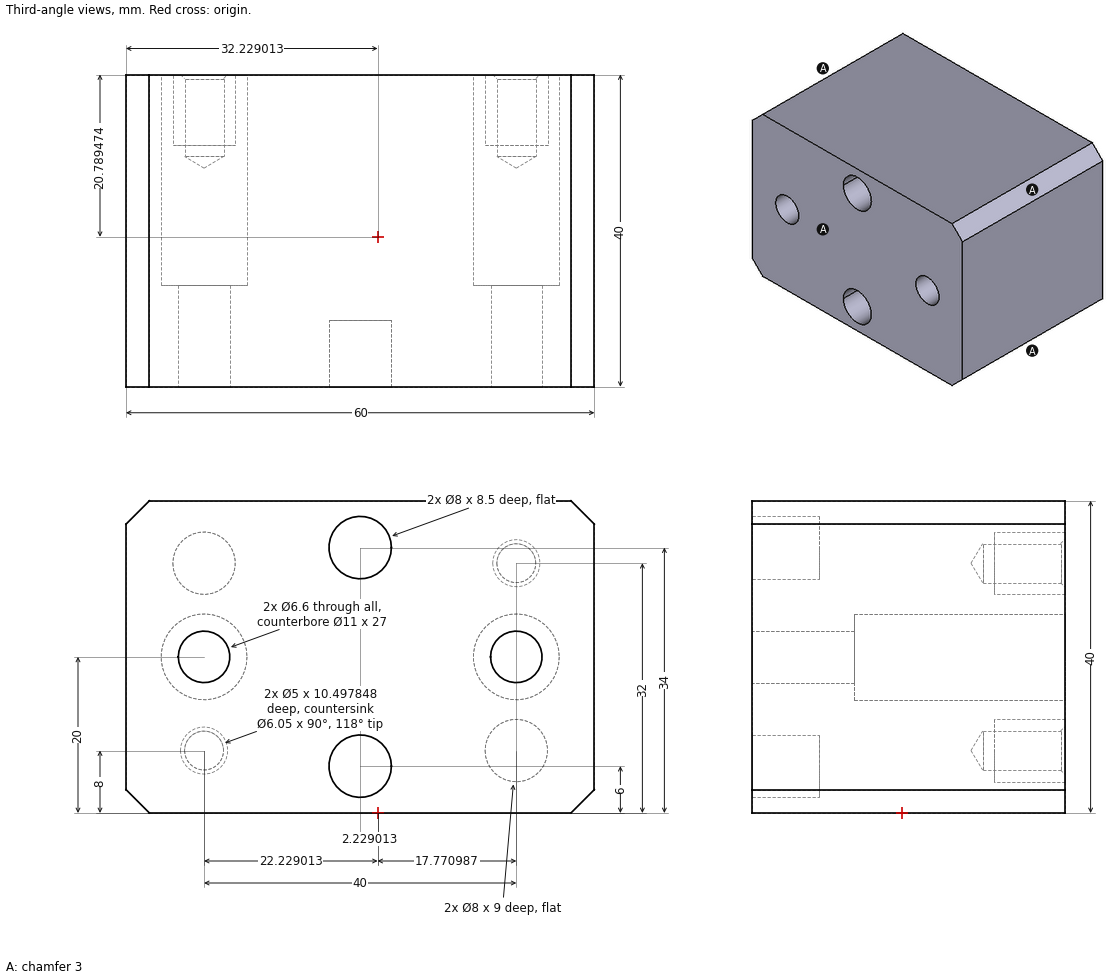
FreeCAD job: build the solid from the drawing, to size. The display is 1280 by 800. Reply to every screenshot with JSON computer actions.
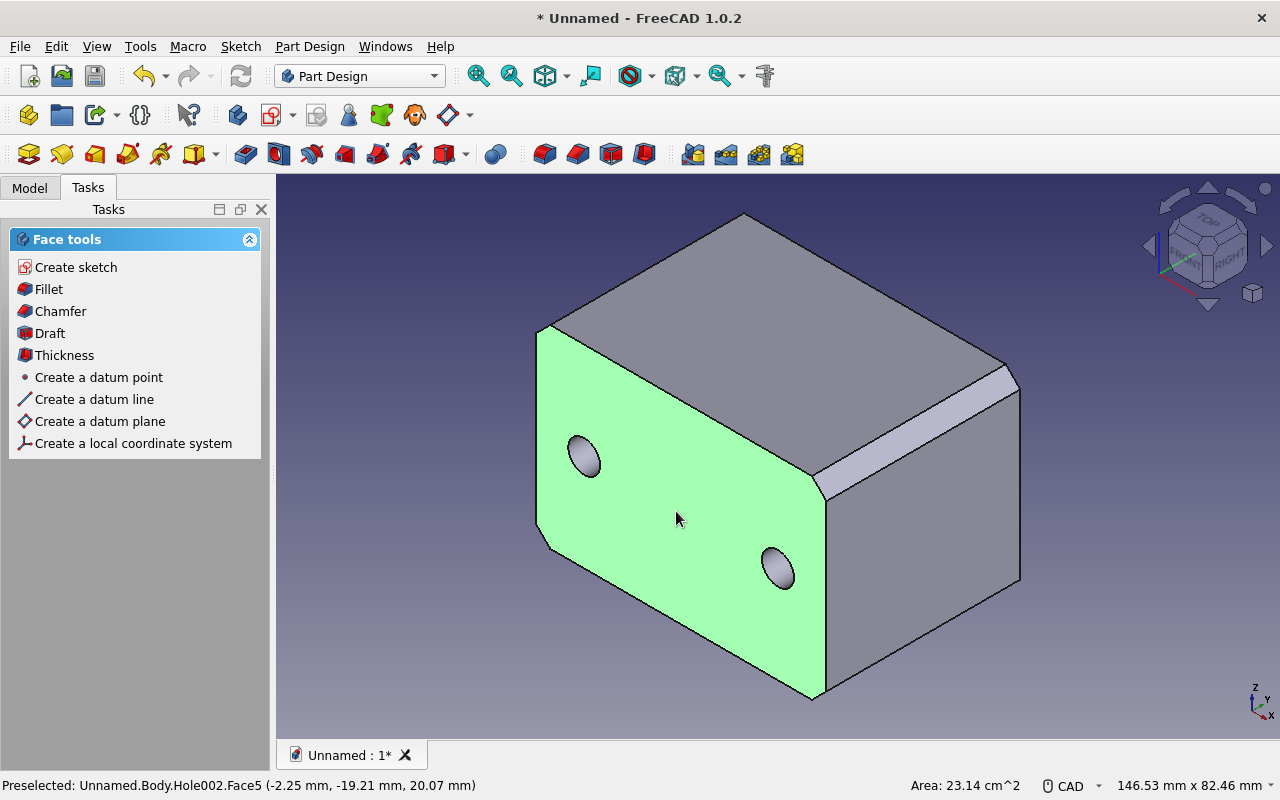
{"action": "left_click", "coordinate": [270, 116]}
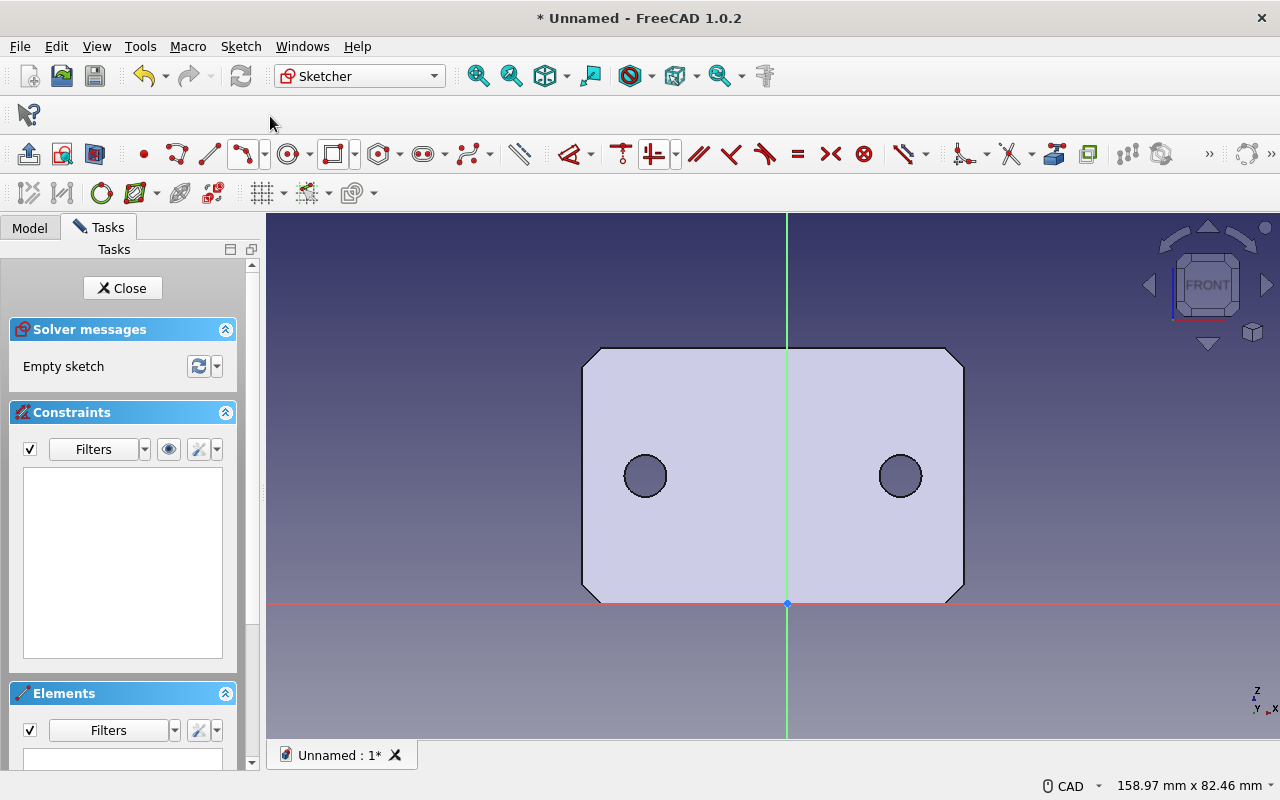
{"action": "scroll", "coordinate": [912, 495], "scroll_direction": "up", "scroll_amount": 2}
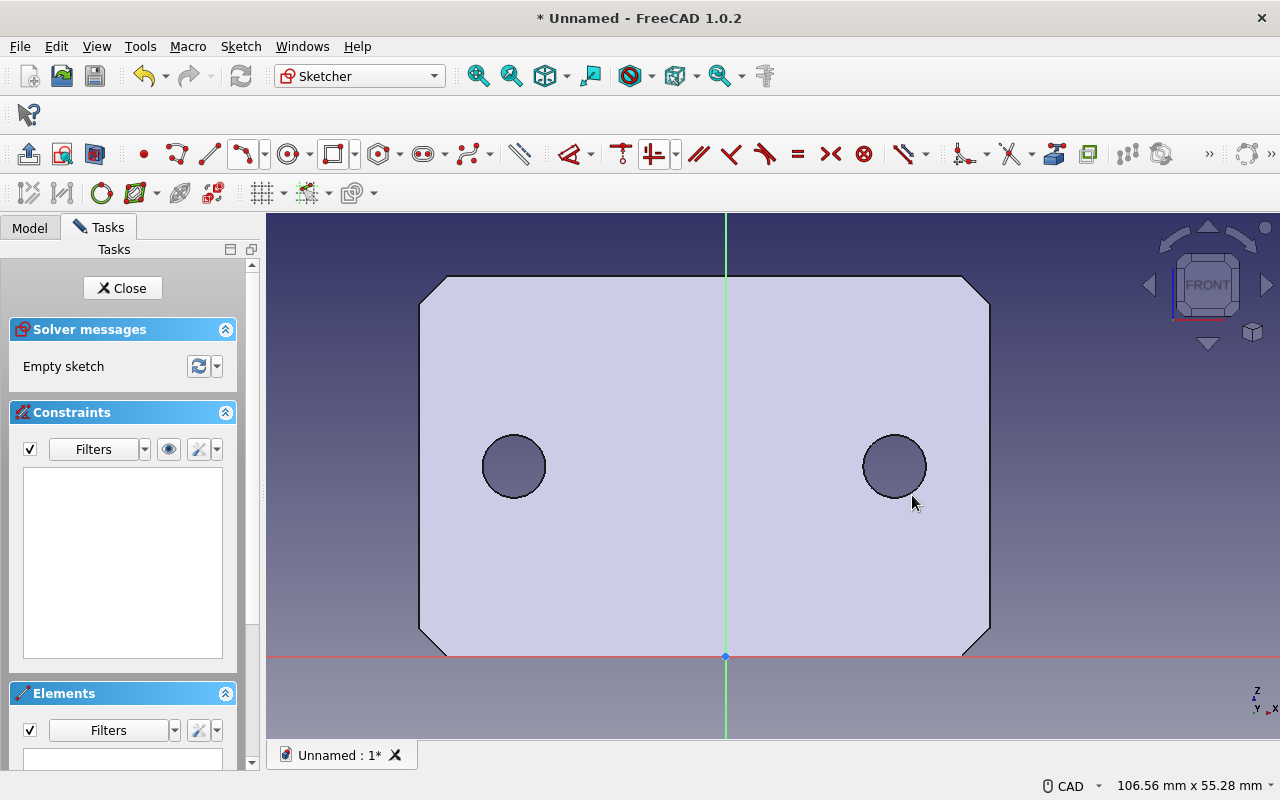
{"action": "left_click", "coordinate": [288, 154]}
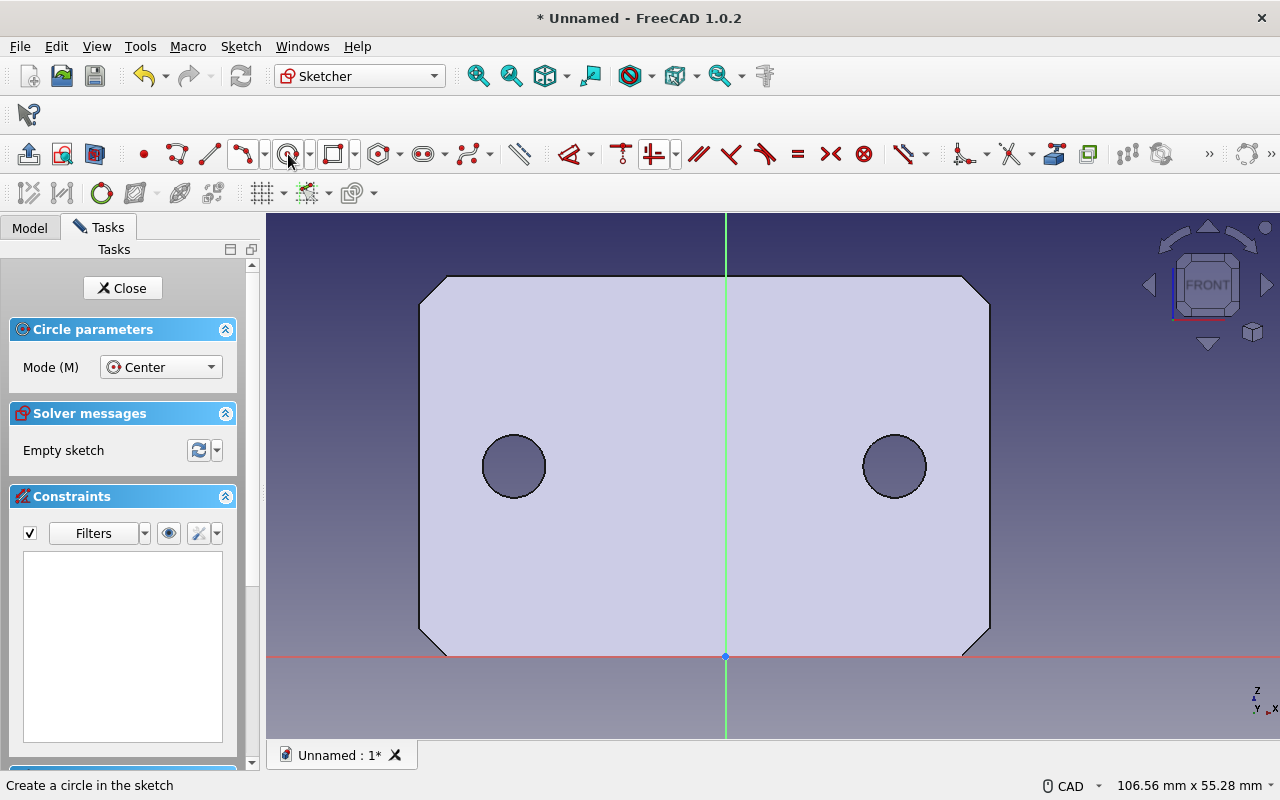
{"action": "left_click", "coordinate": [704, 333]}
{"action": "mouse_move", "coordinate": [677, 306]}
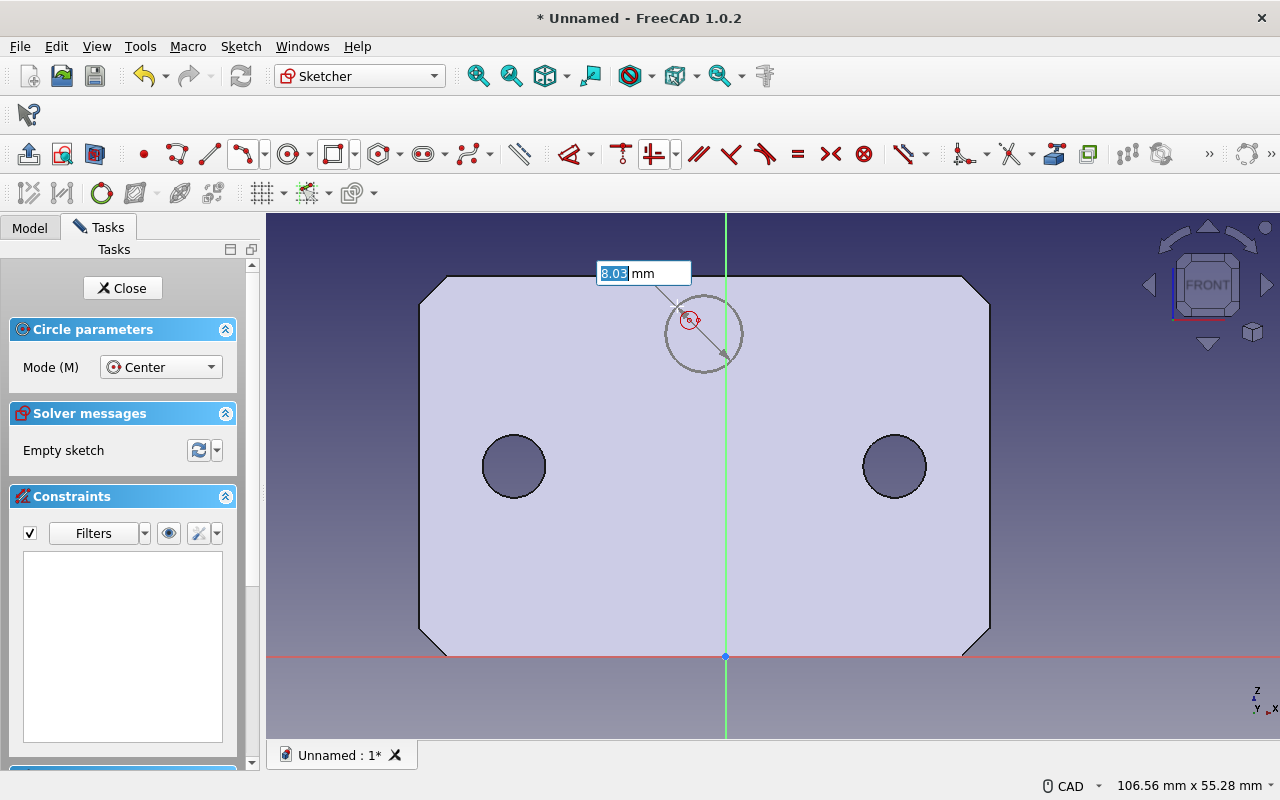
{"action": "type", "text": "8"}
{"action": "key", "text": "Return"}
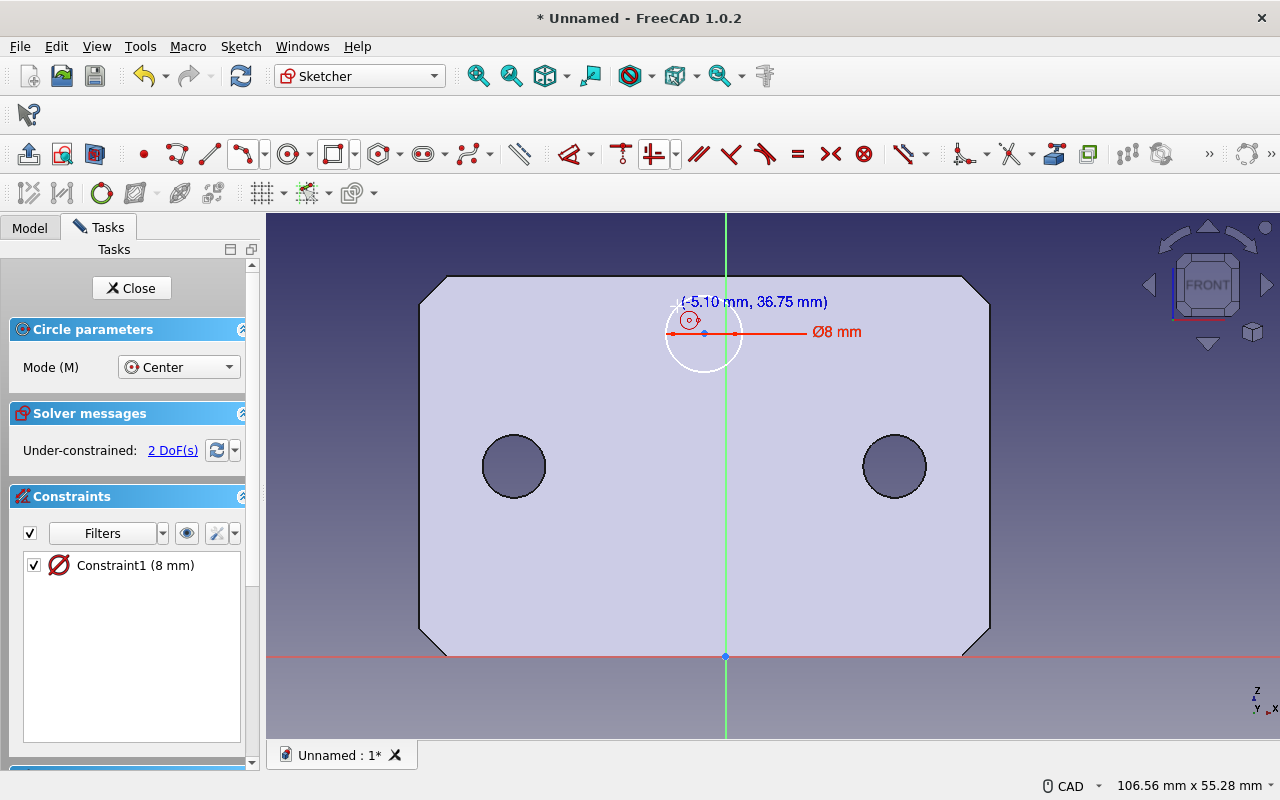
{"action": "left_click", "coordinate": [704, 600]}
{"action": "mouse_move", "coordinate": [677, 573]}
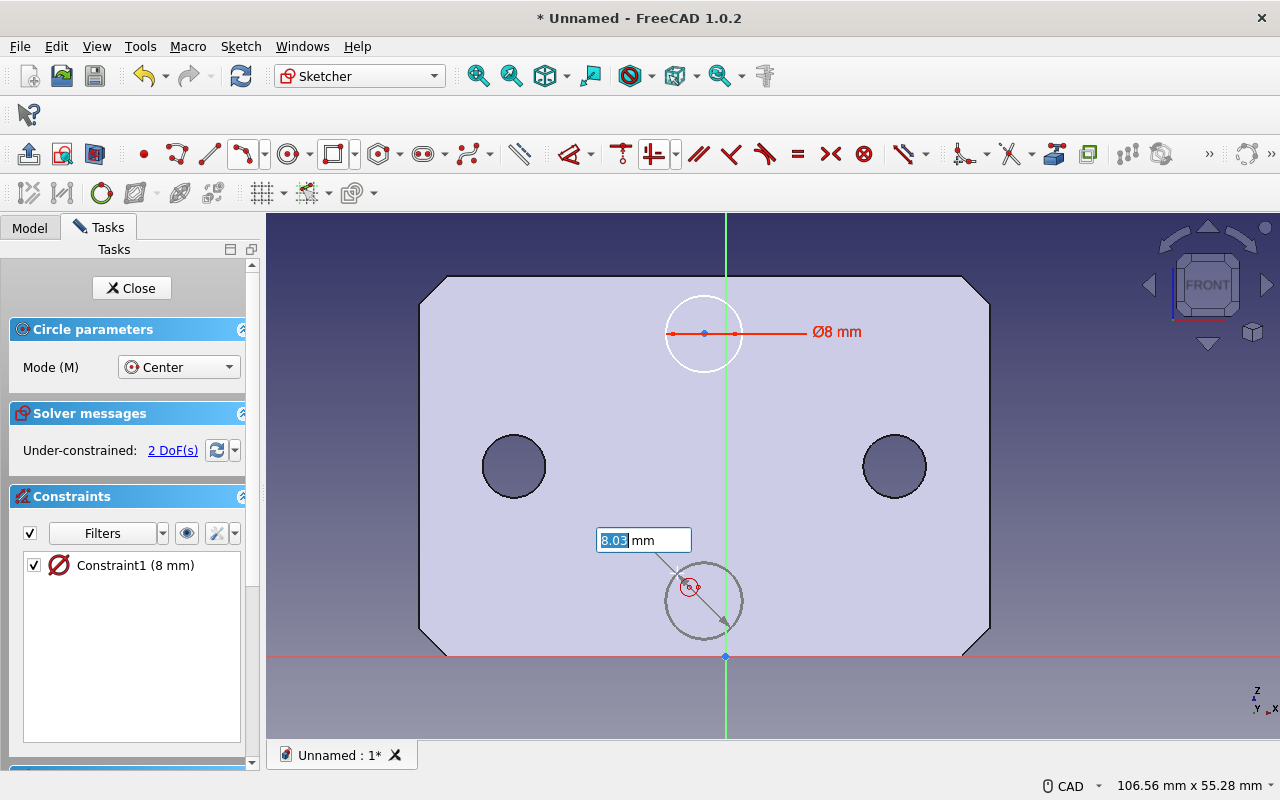
{"action": "type", "text": "8"}
{"action": "key", "text": "Return"}
{"action": "key", "text": "Escape"}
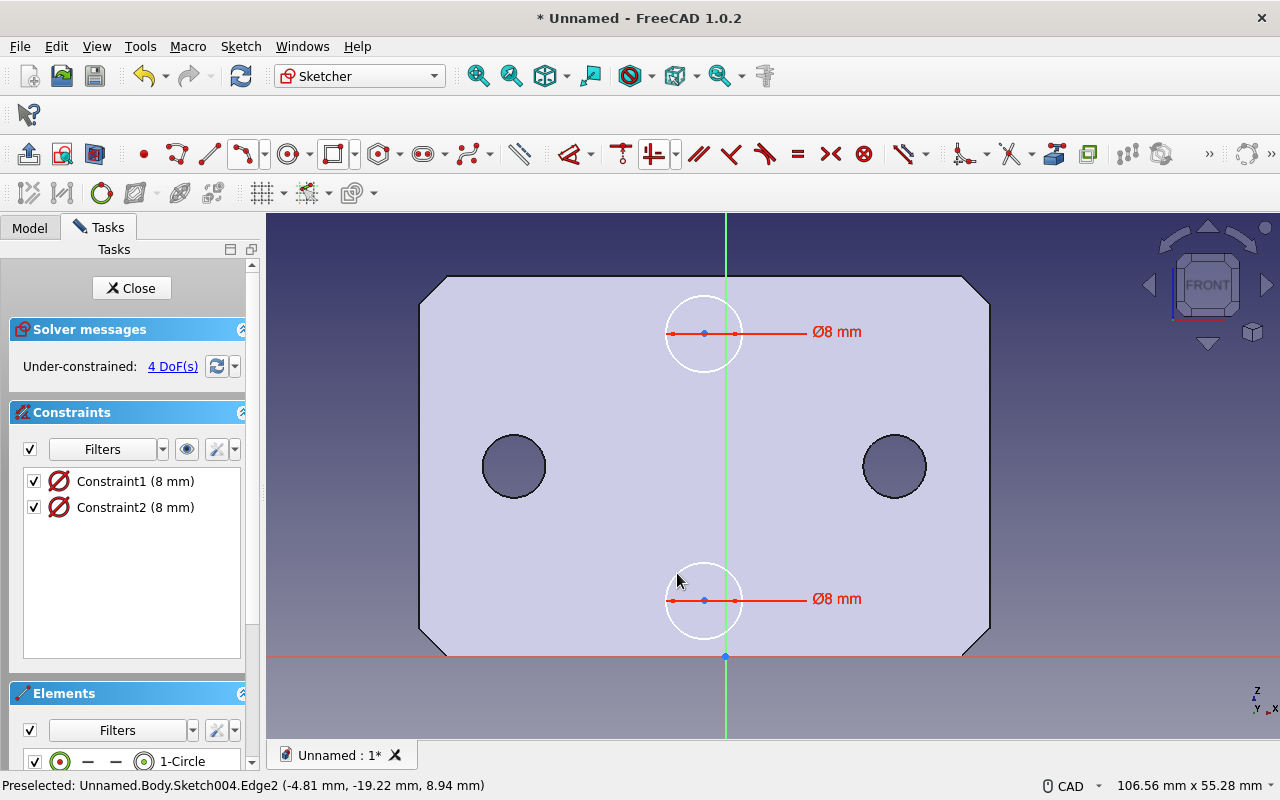
{"action": "key", "text": "d"}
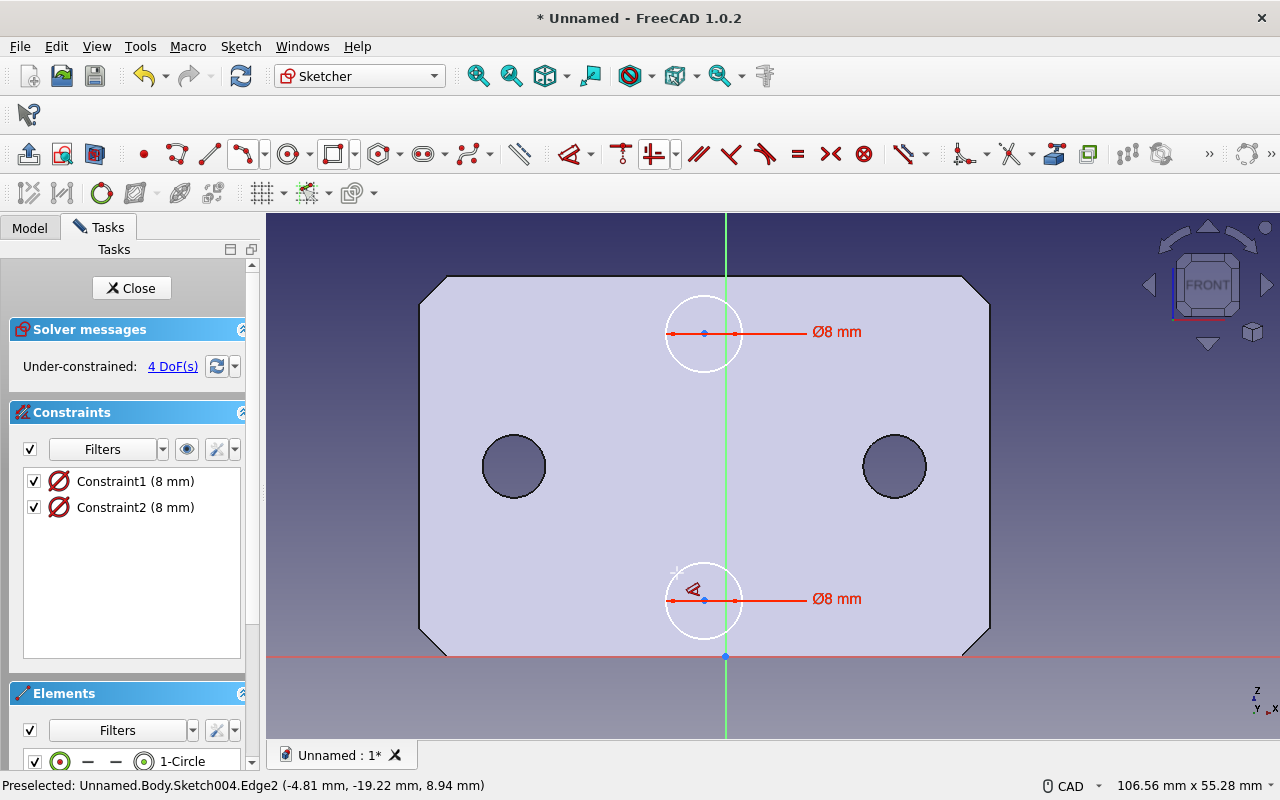
{"action": "left_click", "coordinate": [704, 601]}
{"action": "left_click", "coordinate": [760, 629]}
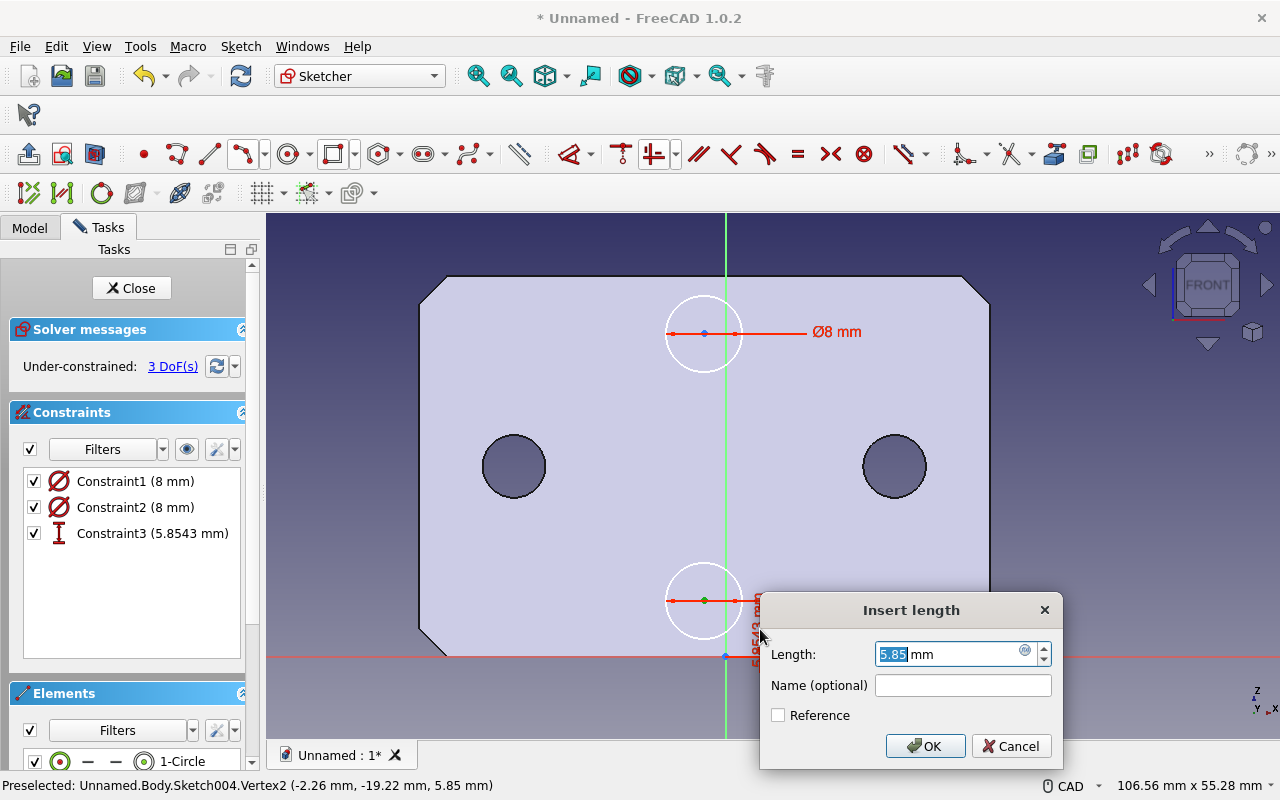
{"action": "type", "text": "6"}
{"action": "key", "text": "Return"}